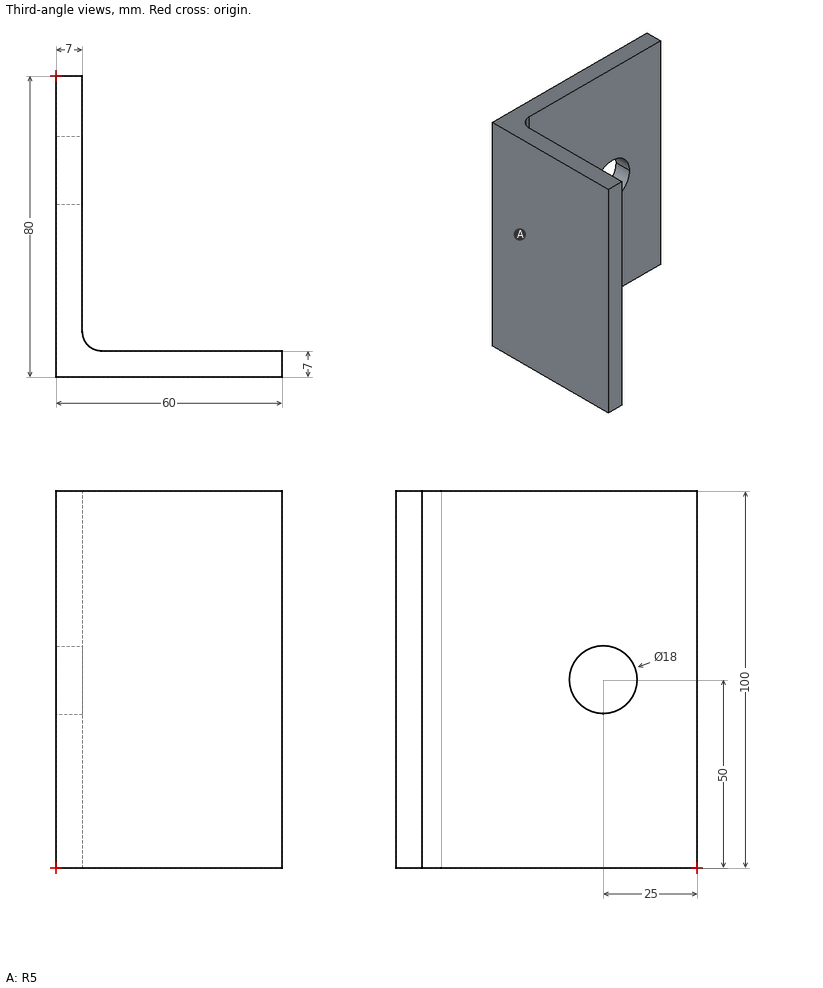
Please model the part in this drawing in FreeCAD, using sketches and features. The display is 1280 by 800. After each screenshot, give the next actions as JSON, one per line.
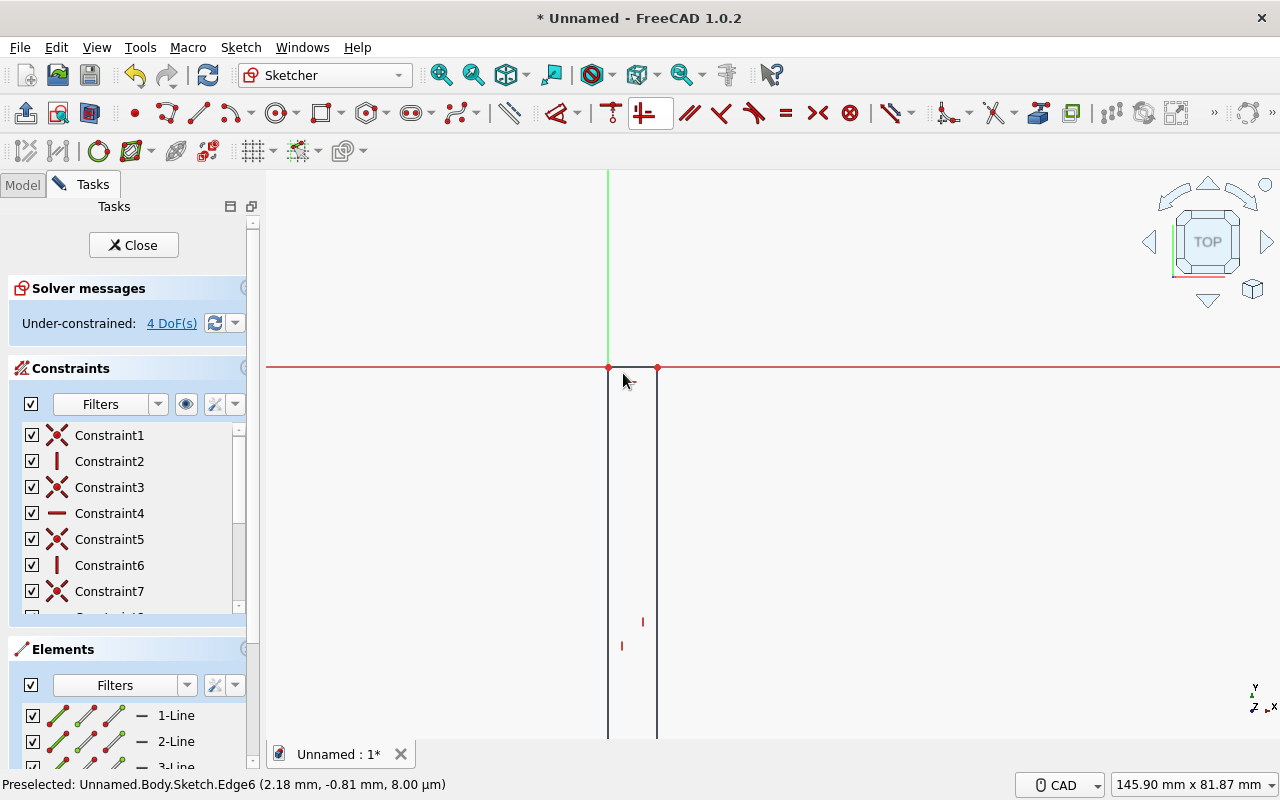
{"action": "left_click", "coordinate": [556, 114]}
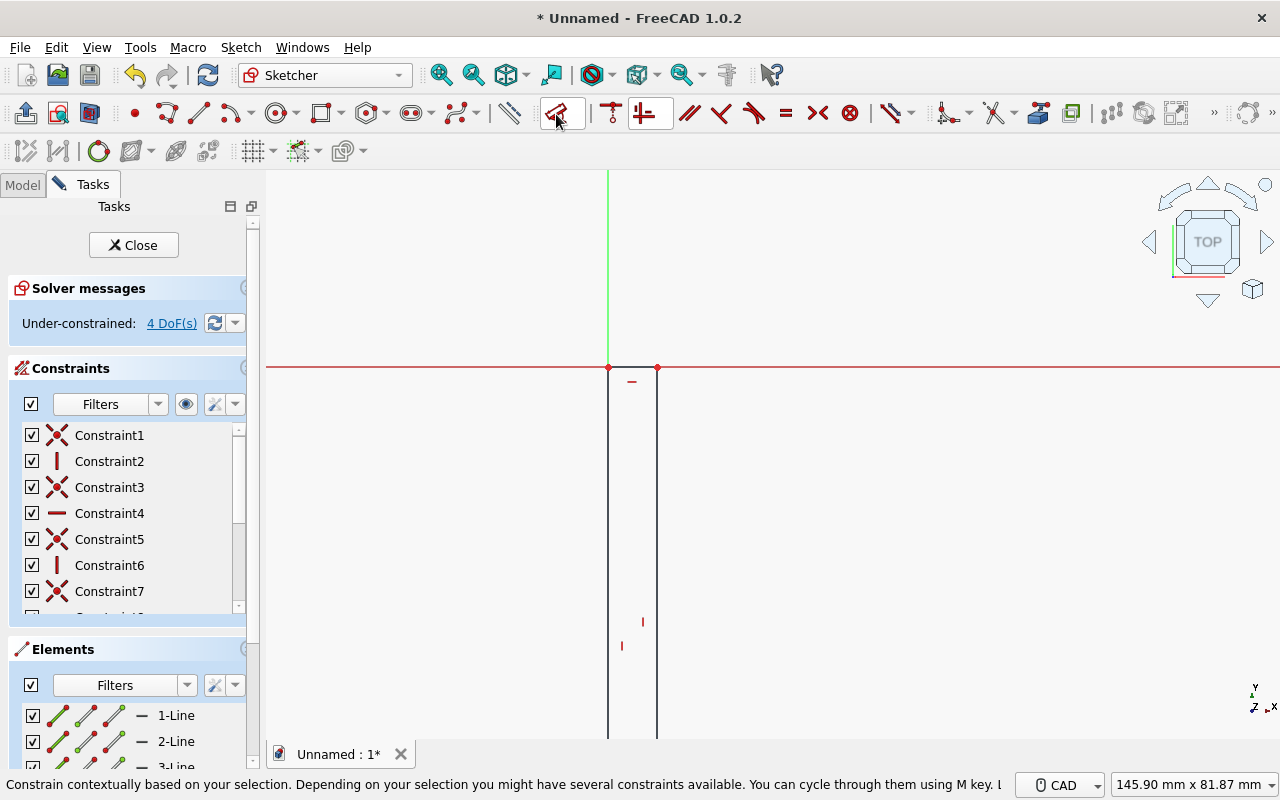
{"action": "scroll", "coordinate": [476, 198], "scroll_direction": "down", "scroll_amount": 2}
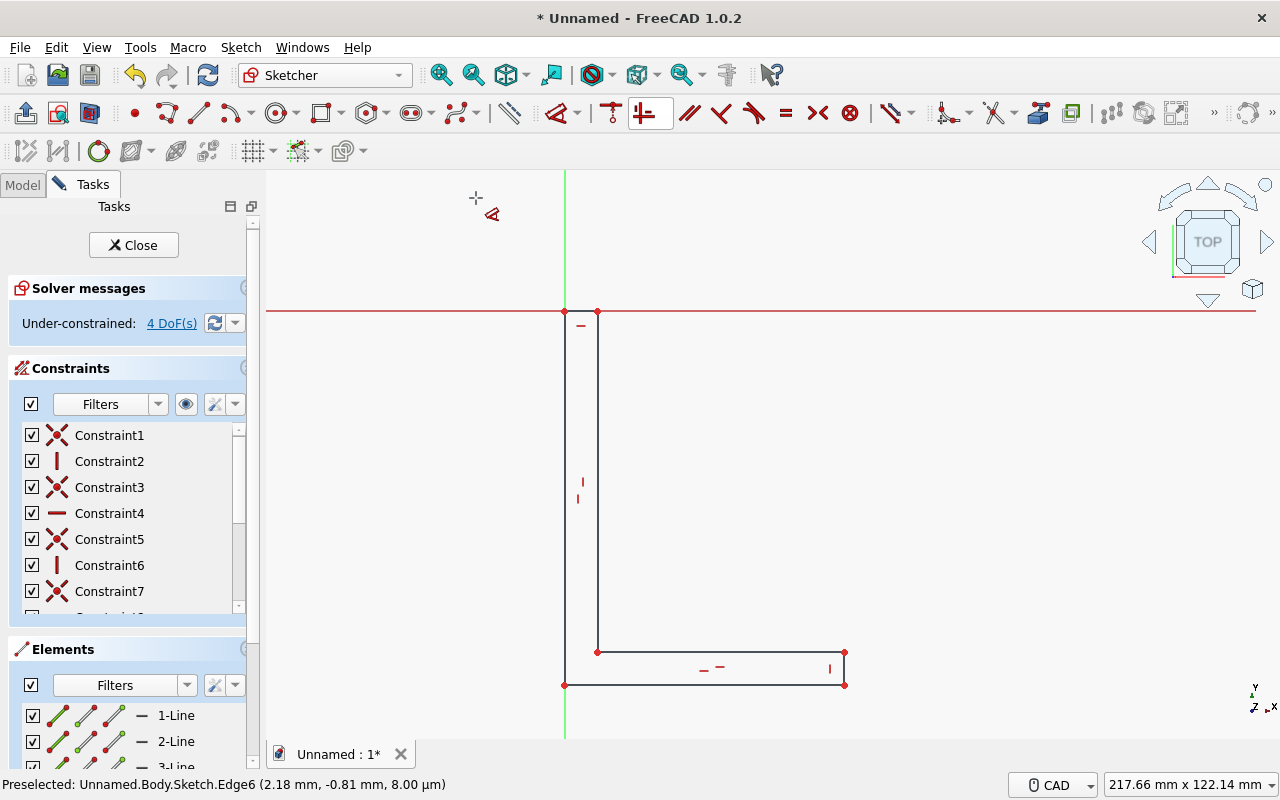
{"action": "scroll", "coordinate": [844, 675], "scroll_direction": "up", "scroll_amount": 2}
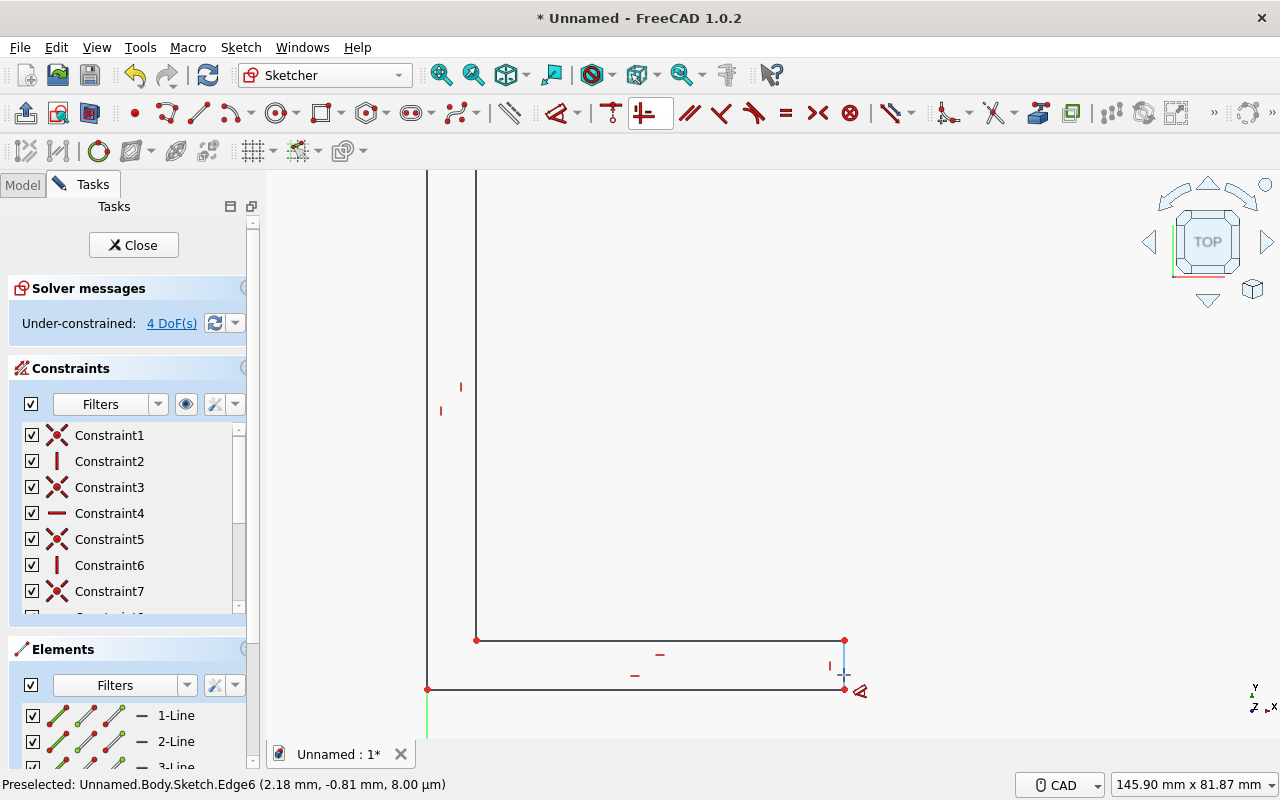
{"action": "left_click", "coordinate": [844, 675]}
{"action": "left_click", "coordinate": [878, 665]}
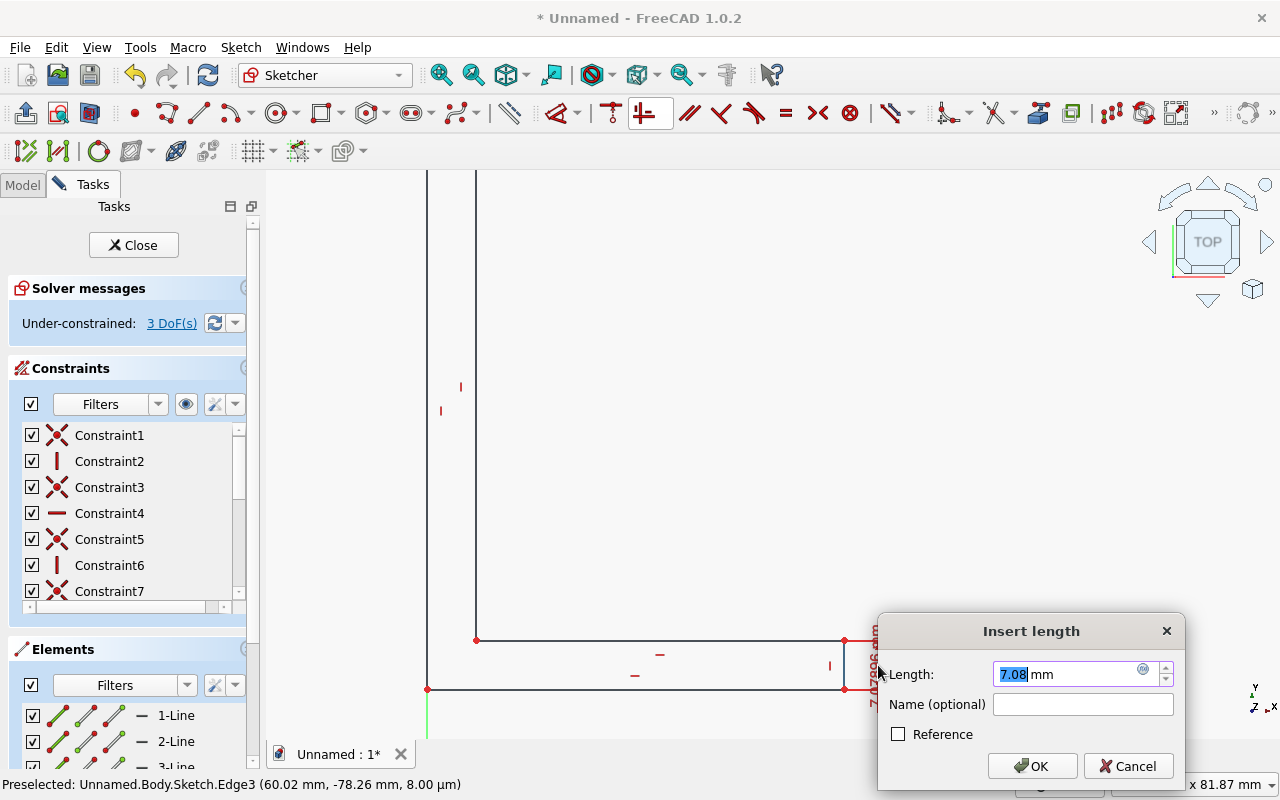
{"action": "type", "text": "7"}
{"action": "key", "text": "Return"}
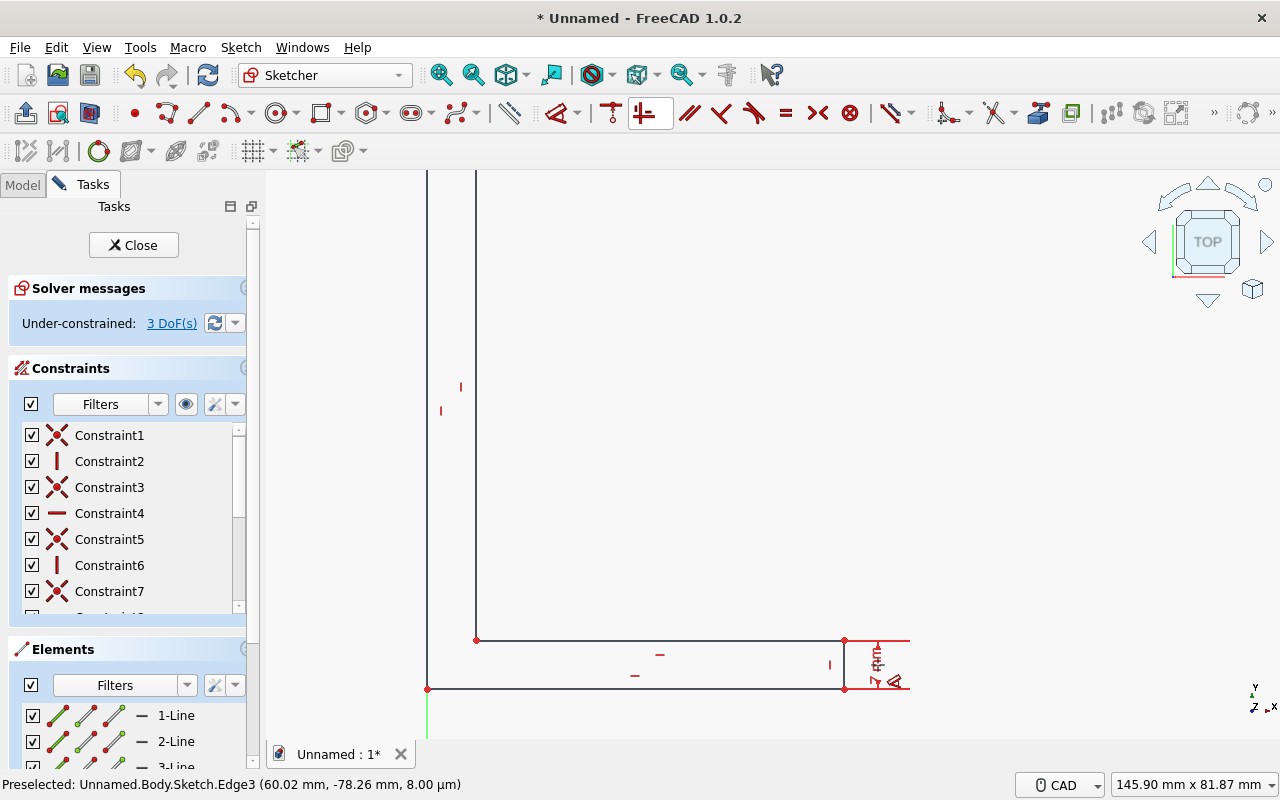
{"action": "scroll", "coordinate": [845, 545], "scroll_direction": "down", "scroll_amount": 2}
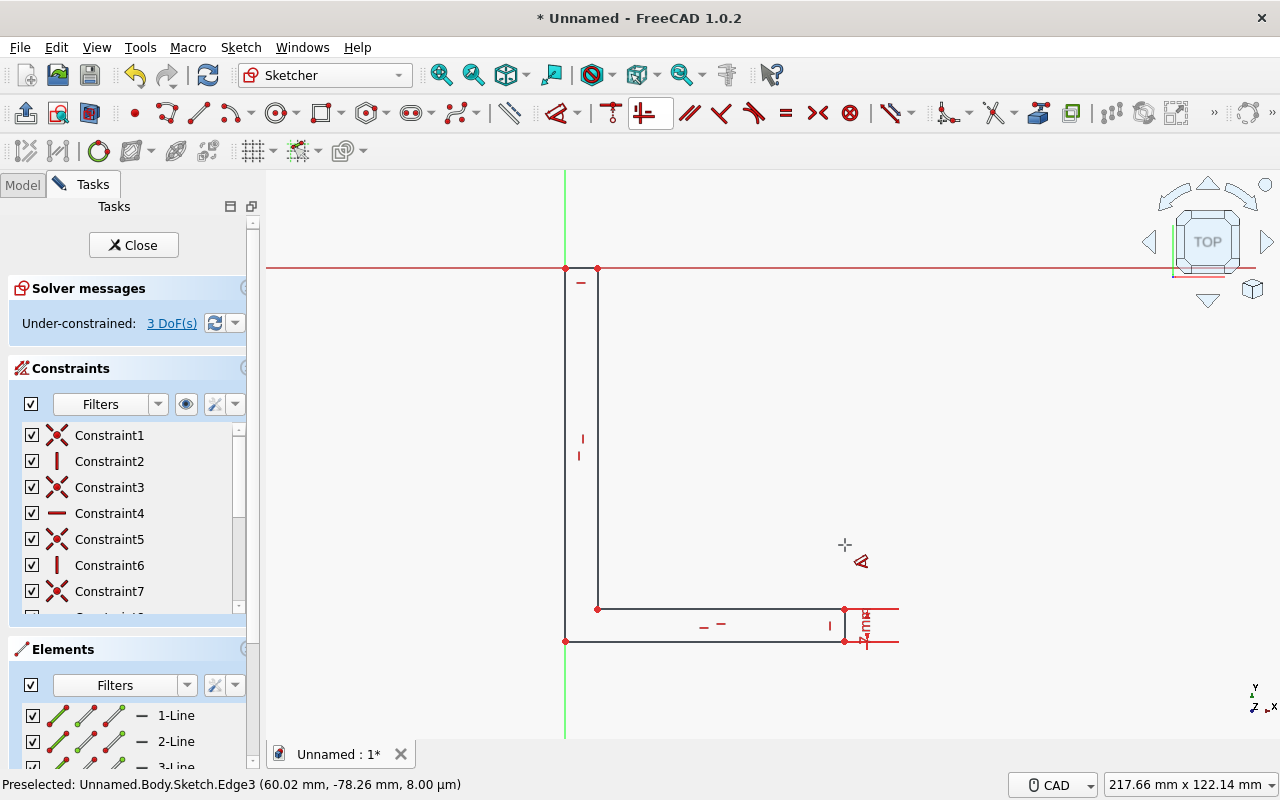
{"action": "scroll", "coordinate": [588, 268], "scroll_direction": "up", "scroll_amount": 2}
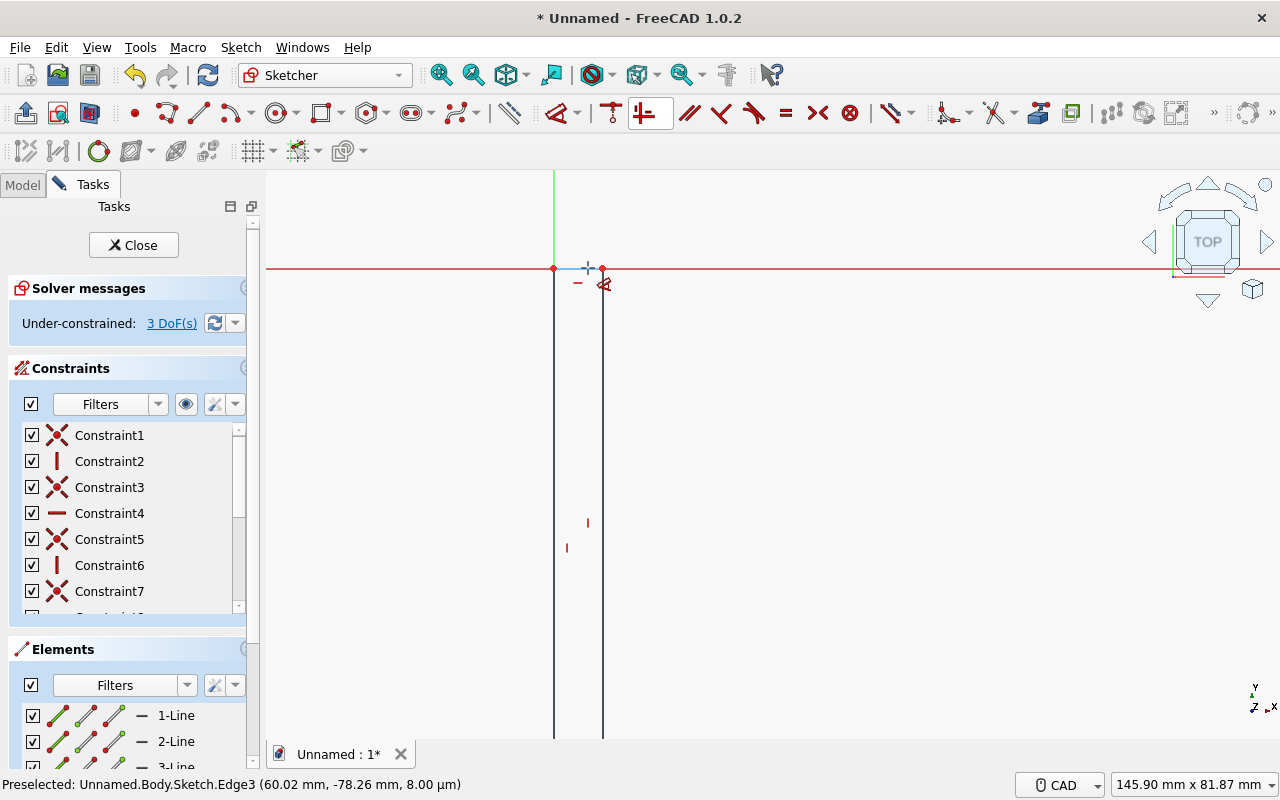
{"action": "left_click", "coordinate": [588, 269]}
{"action": "left_click", "coordinate": [578, 235]}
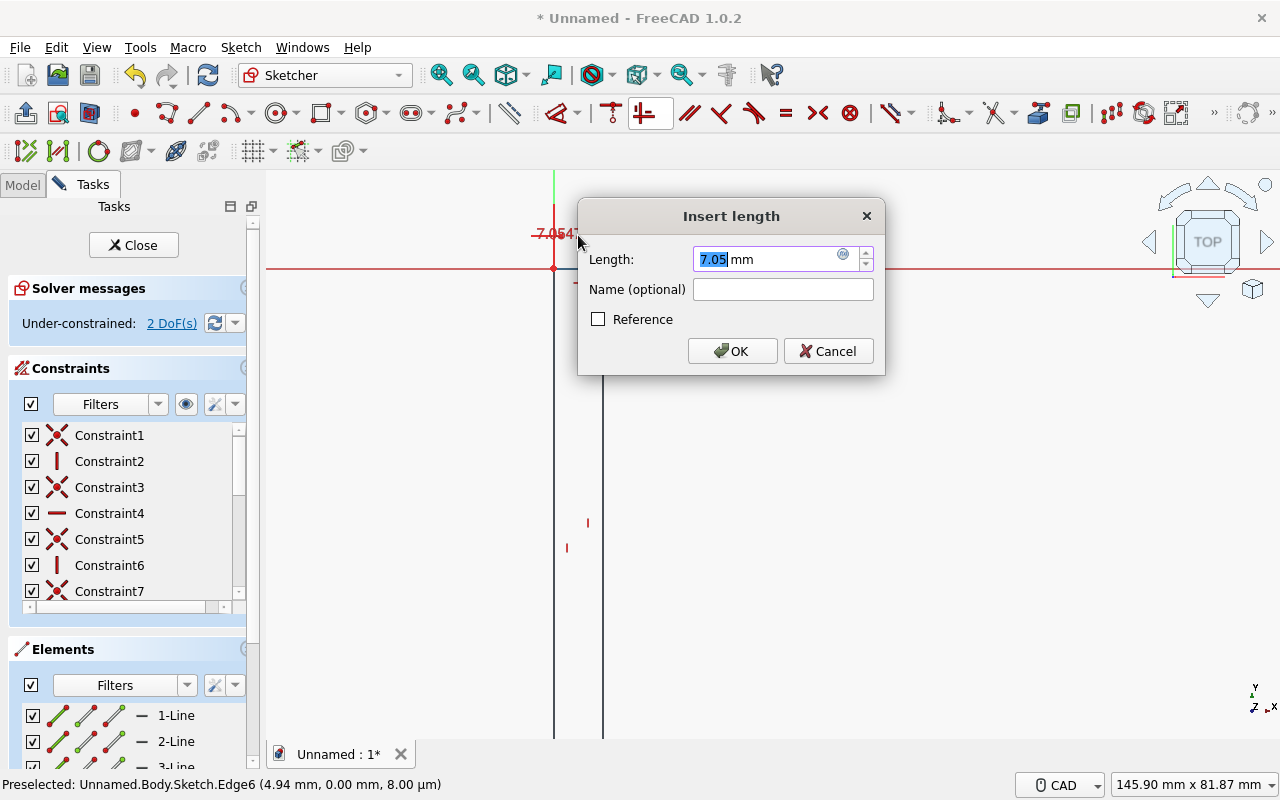
{"action": "type", "text": "7"}
{"action": "key", "text": "Return"}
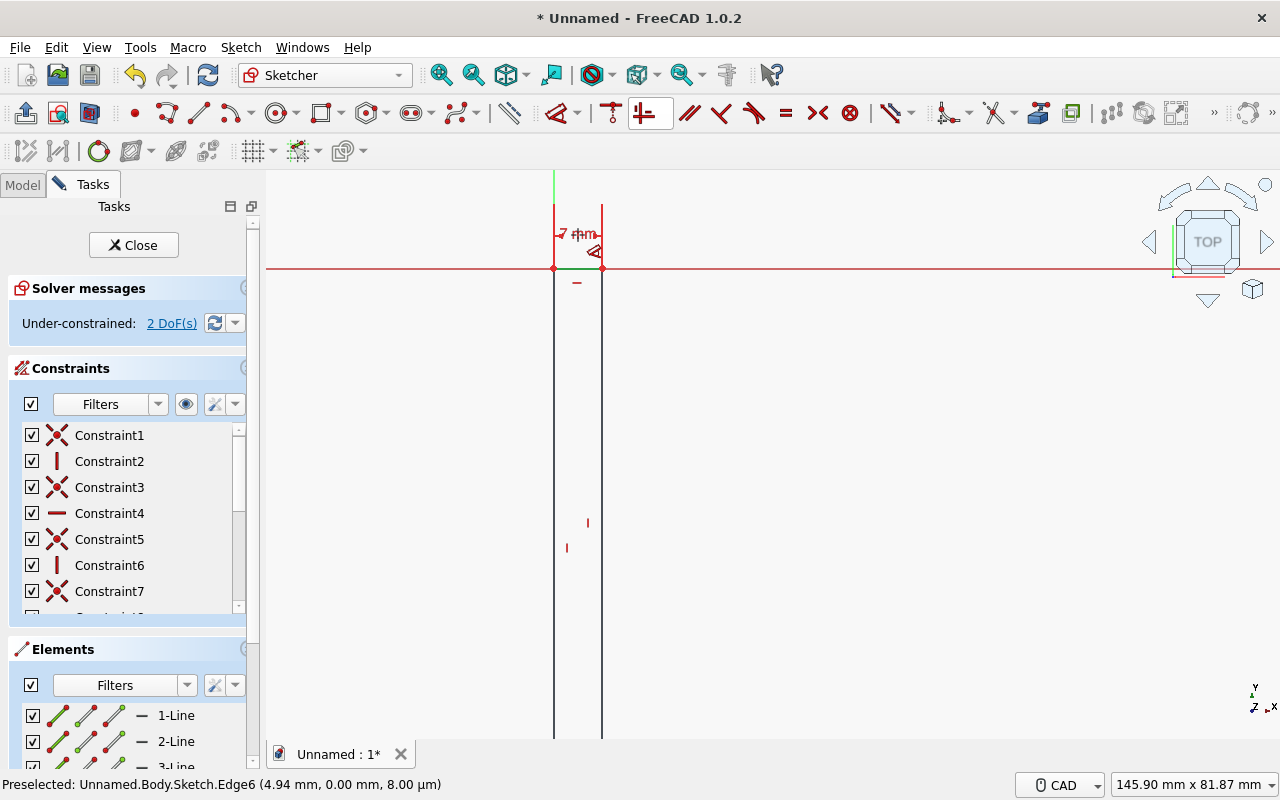
{"action": "left_click", "coordinate": [554, 436]}
{"action": "left_click", "coordinate": [520, 490]}